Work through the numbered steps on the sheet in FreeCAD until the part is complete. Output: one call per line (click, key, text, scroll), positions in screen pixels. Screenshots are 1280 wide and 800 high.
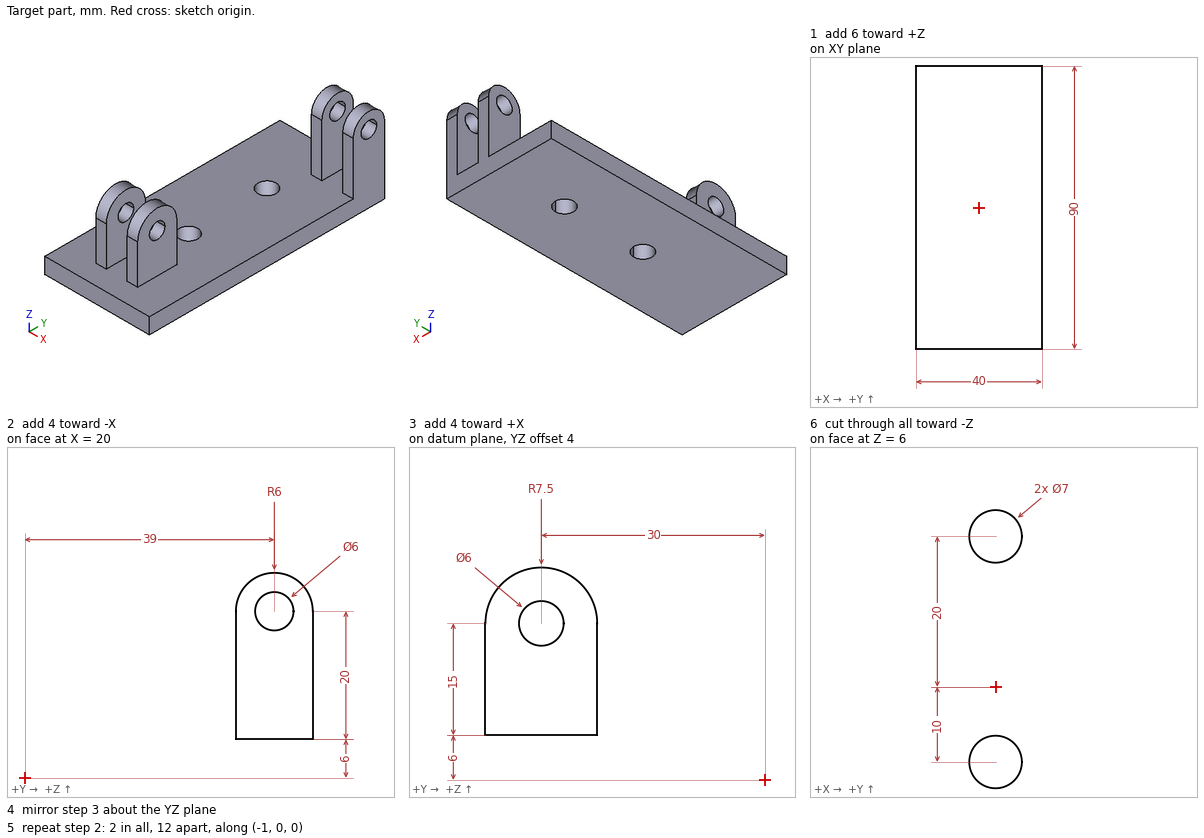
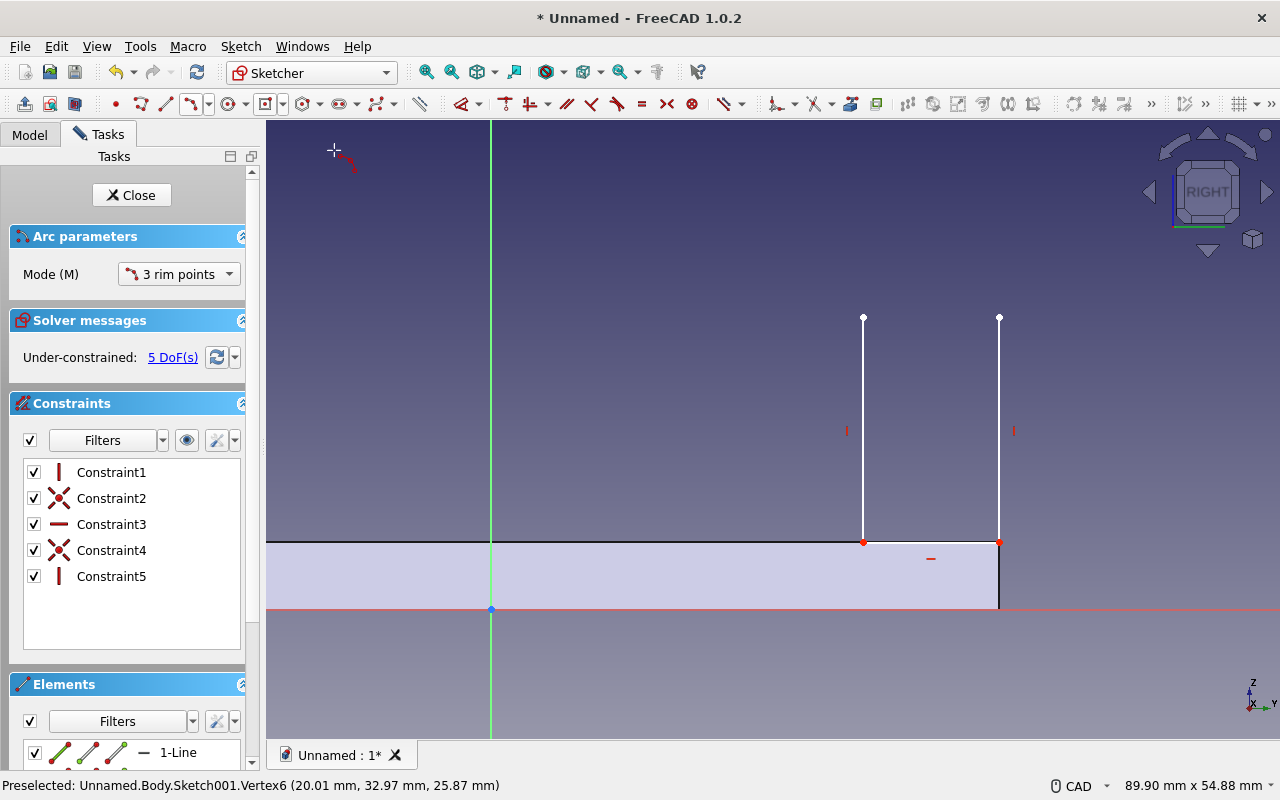
click(863, 318)
click(999, 318)
click(931, 249)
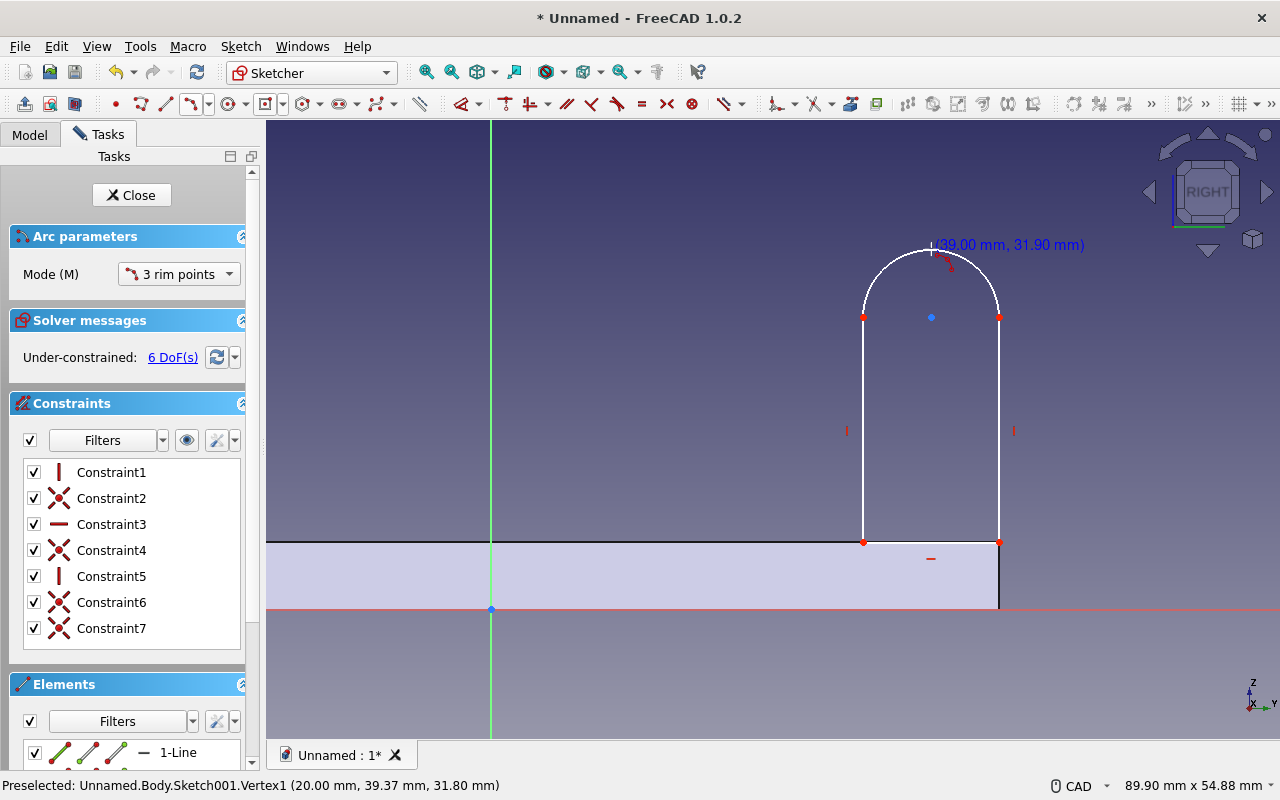
click(228, 104)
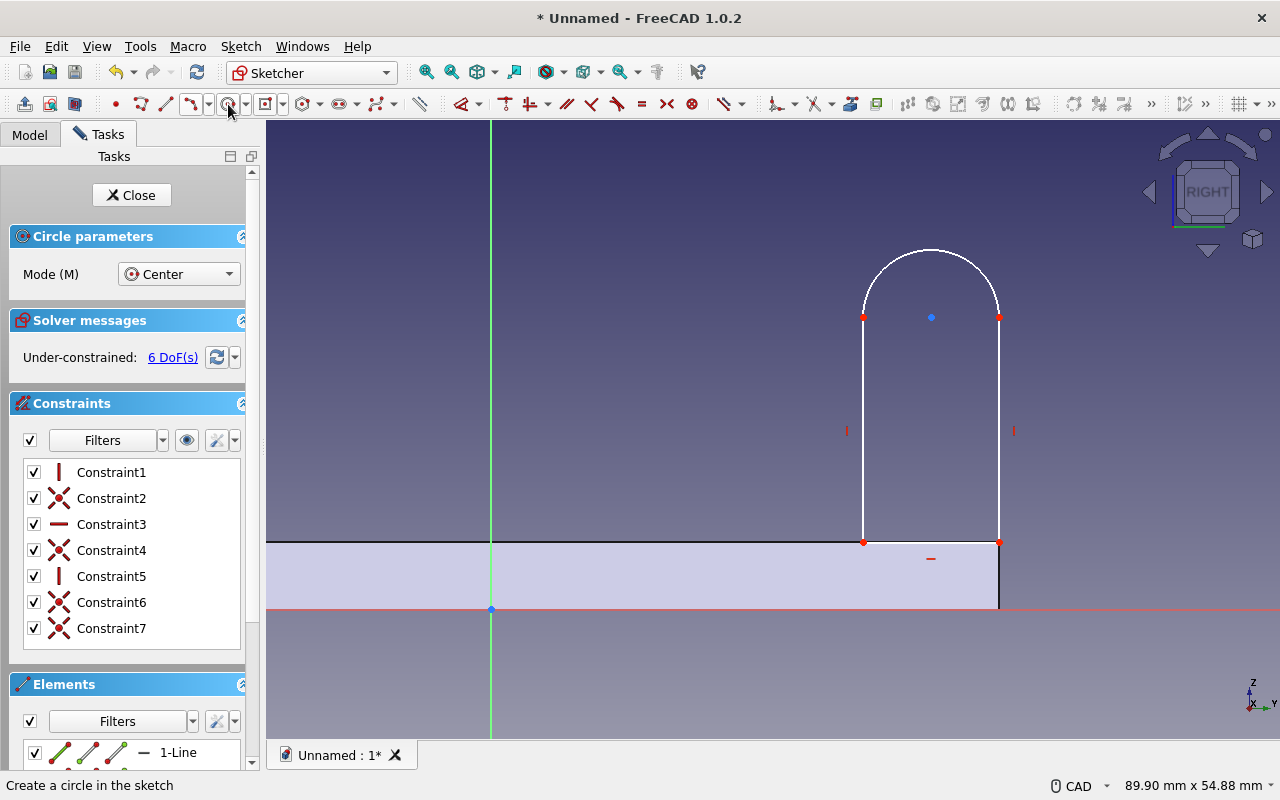
click(931, 317)
move(955, 293)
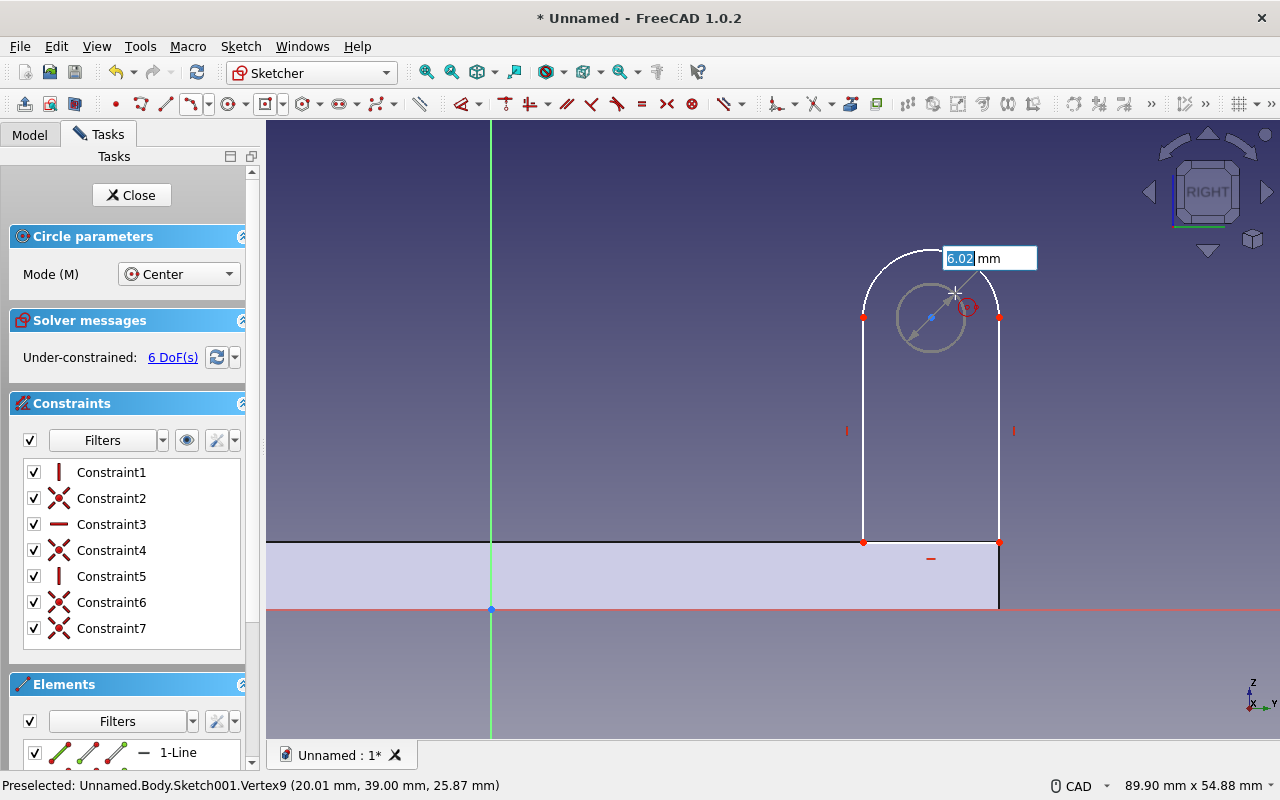
text(6)
key(Return)
key(Escape)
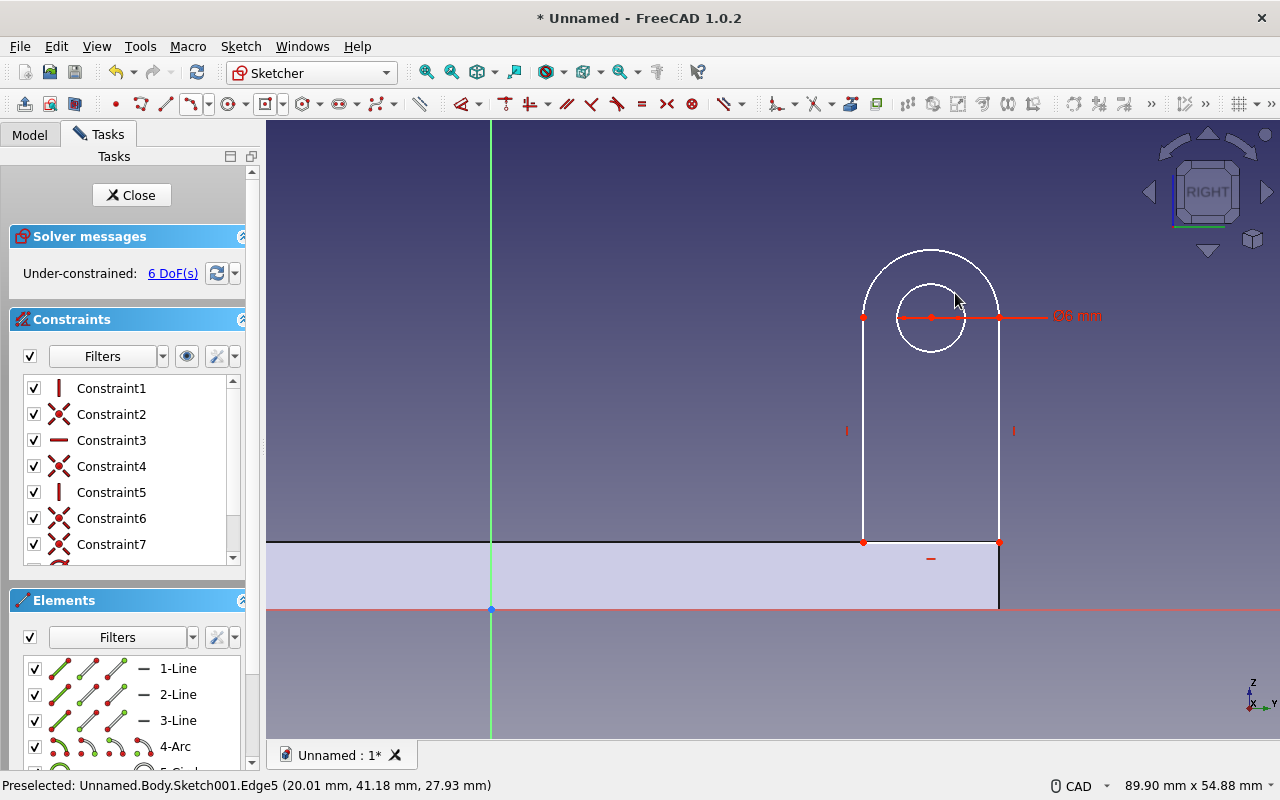
click(999, 386)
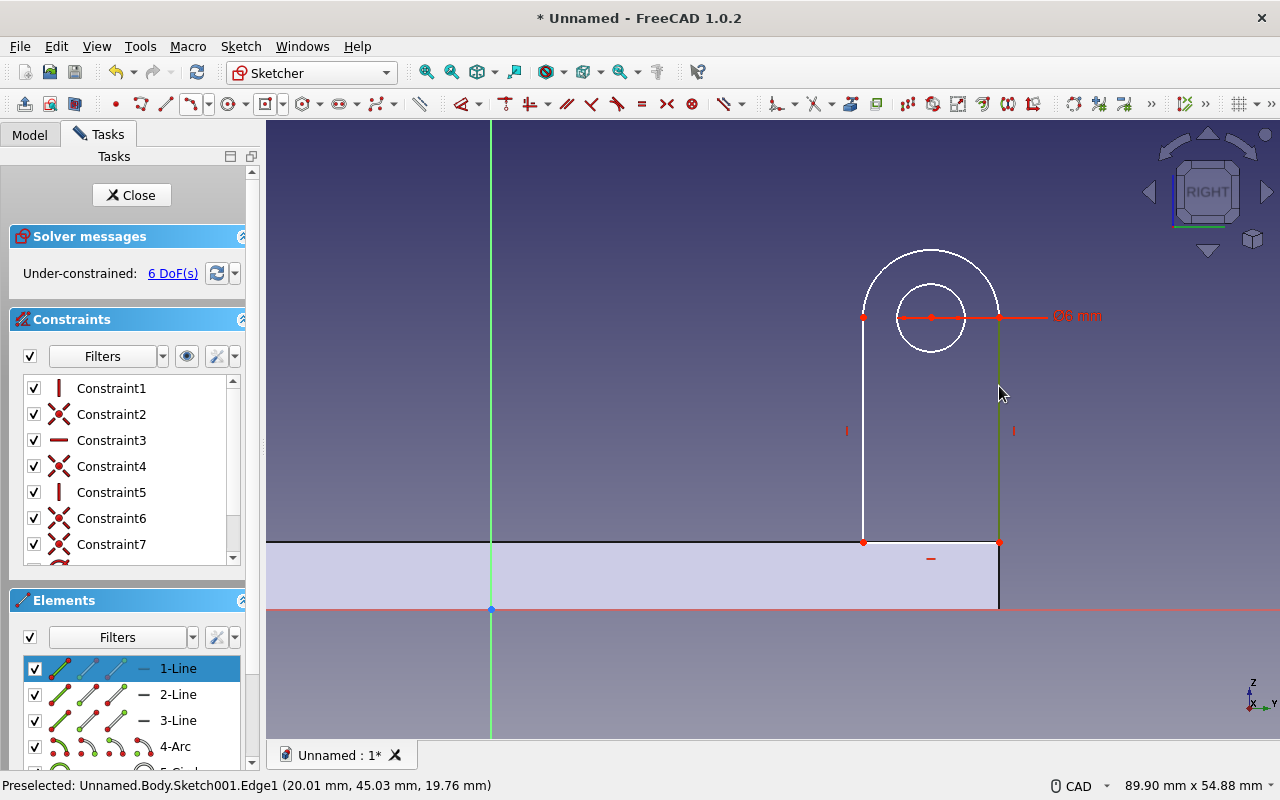
click(971, 263)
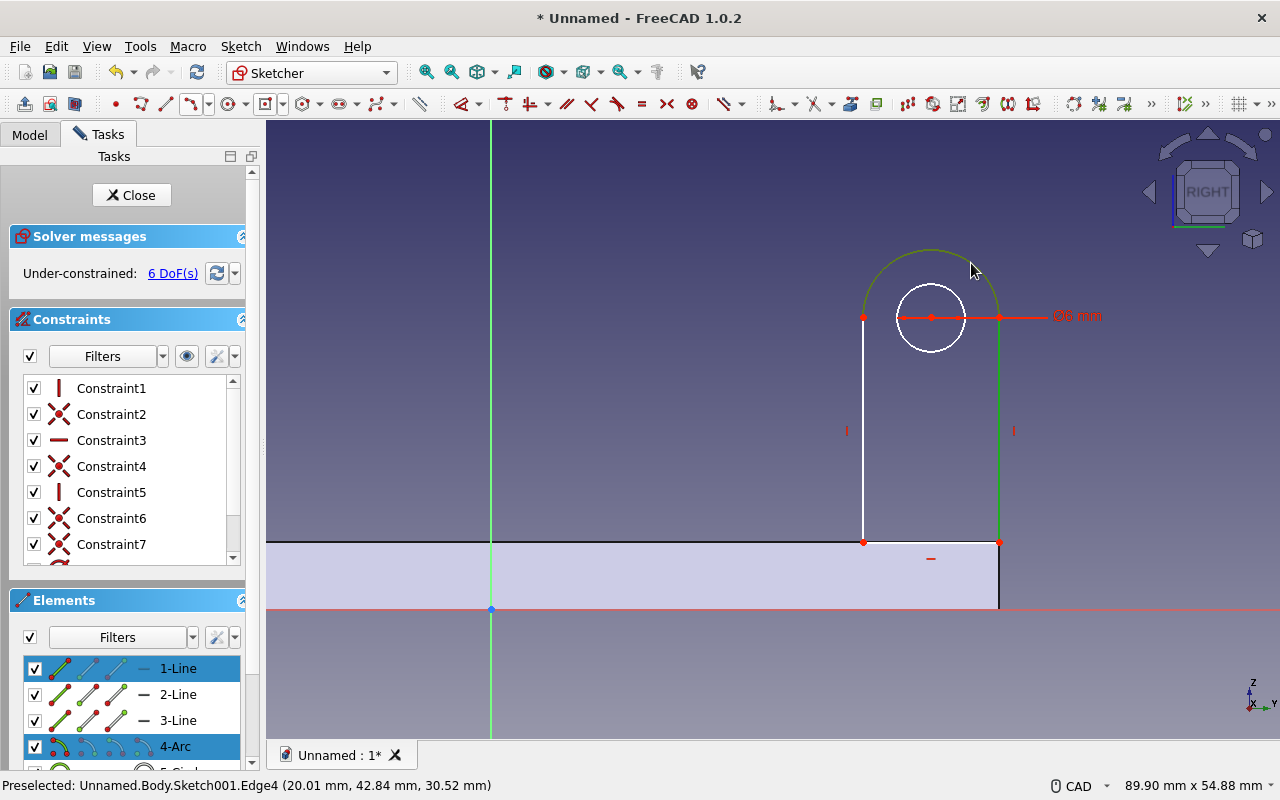
click(617, 104)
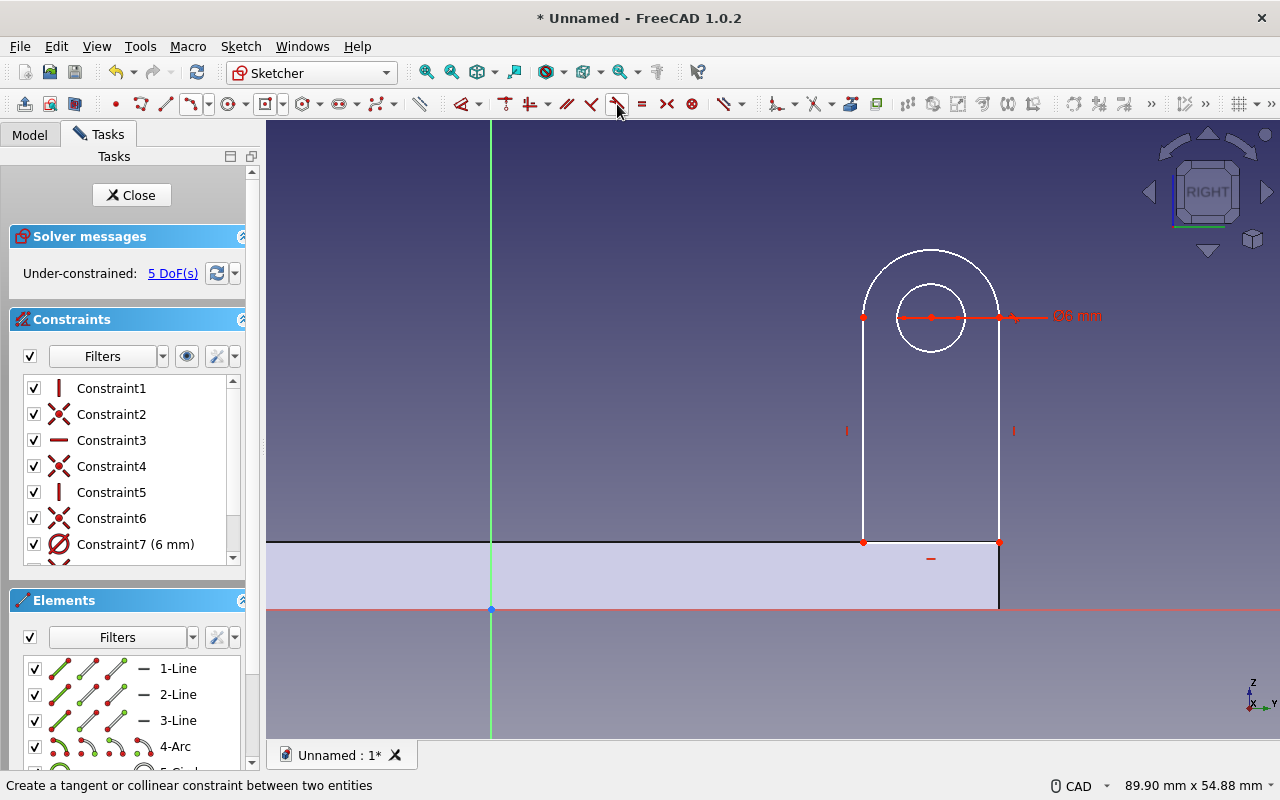
click(863, 475)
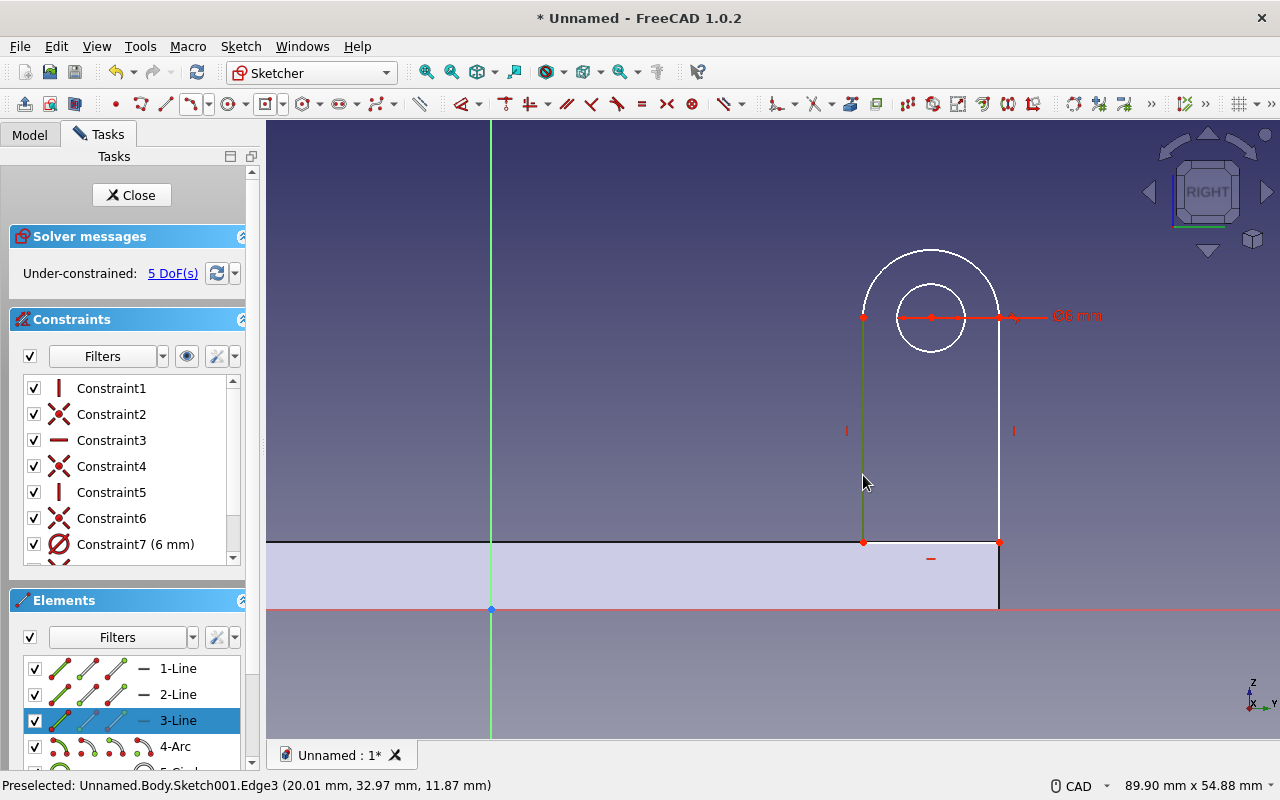
click(971, 263)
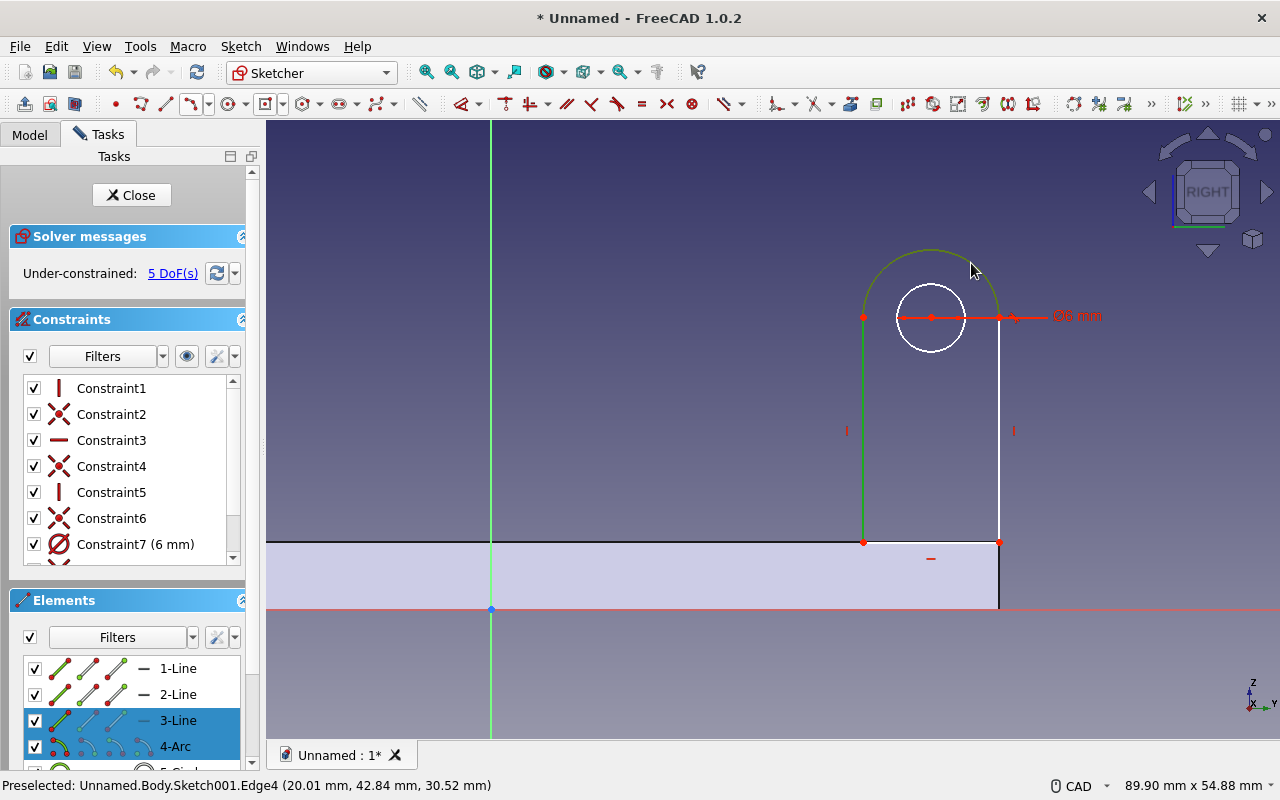
click(617, 104)